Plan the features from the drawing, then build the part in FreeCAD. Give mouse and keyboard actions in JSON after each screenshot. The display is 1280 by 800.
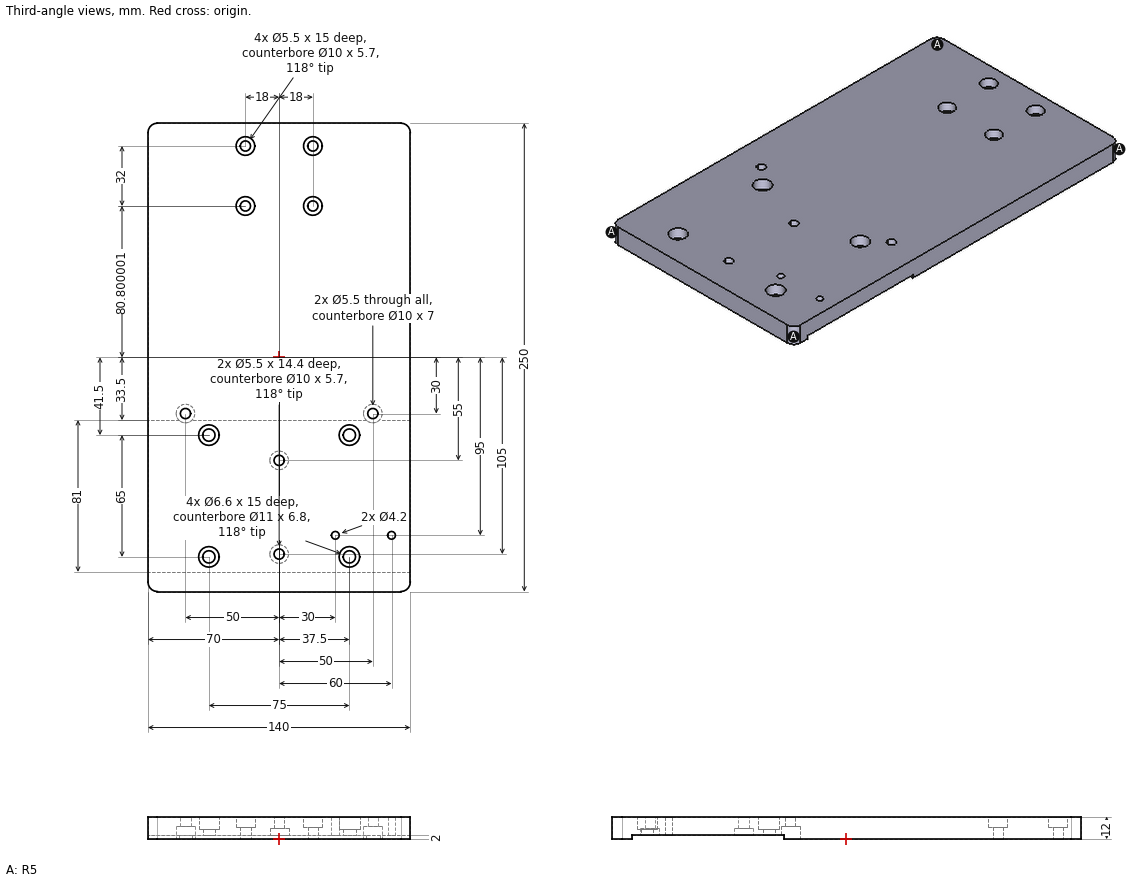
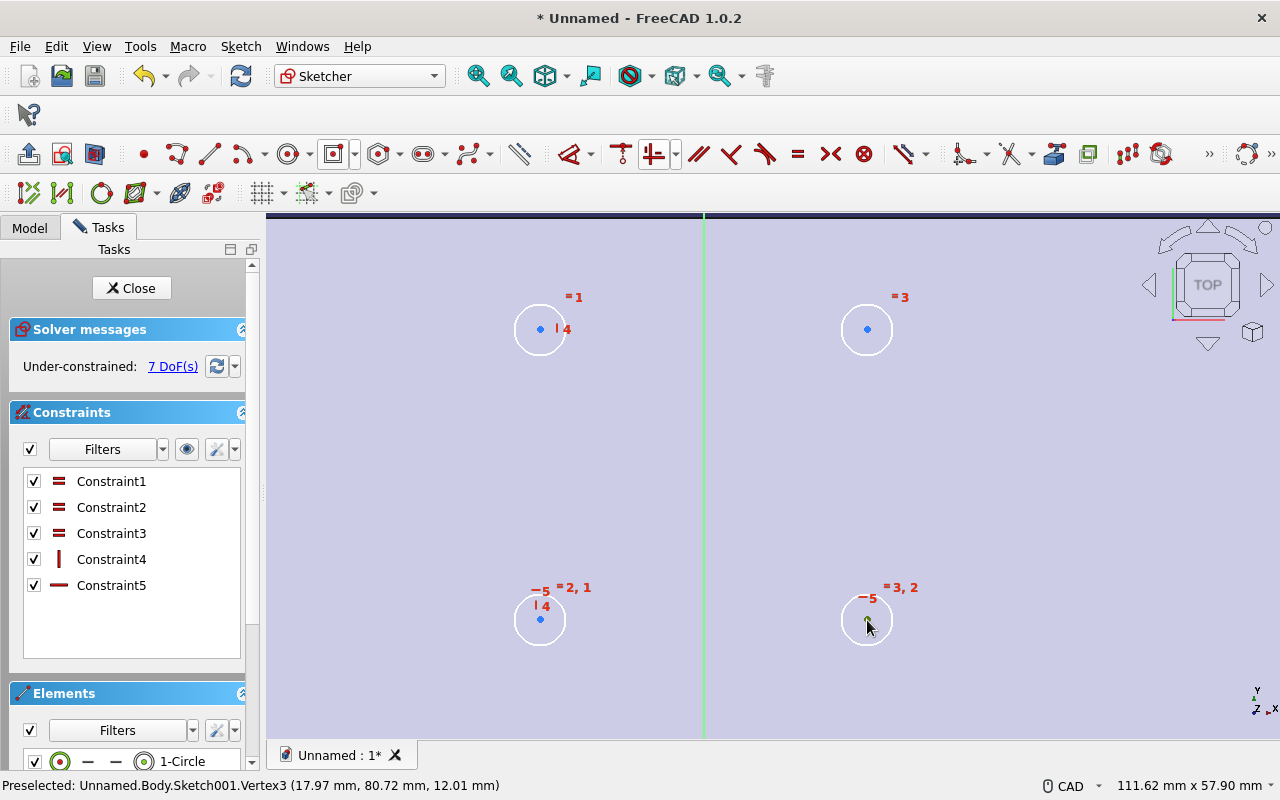
{"action": "left_click", "coordinate": [867, 330]}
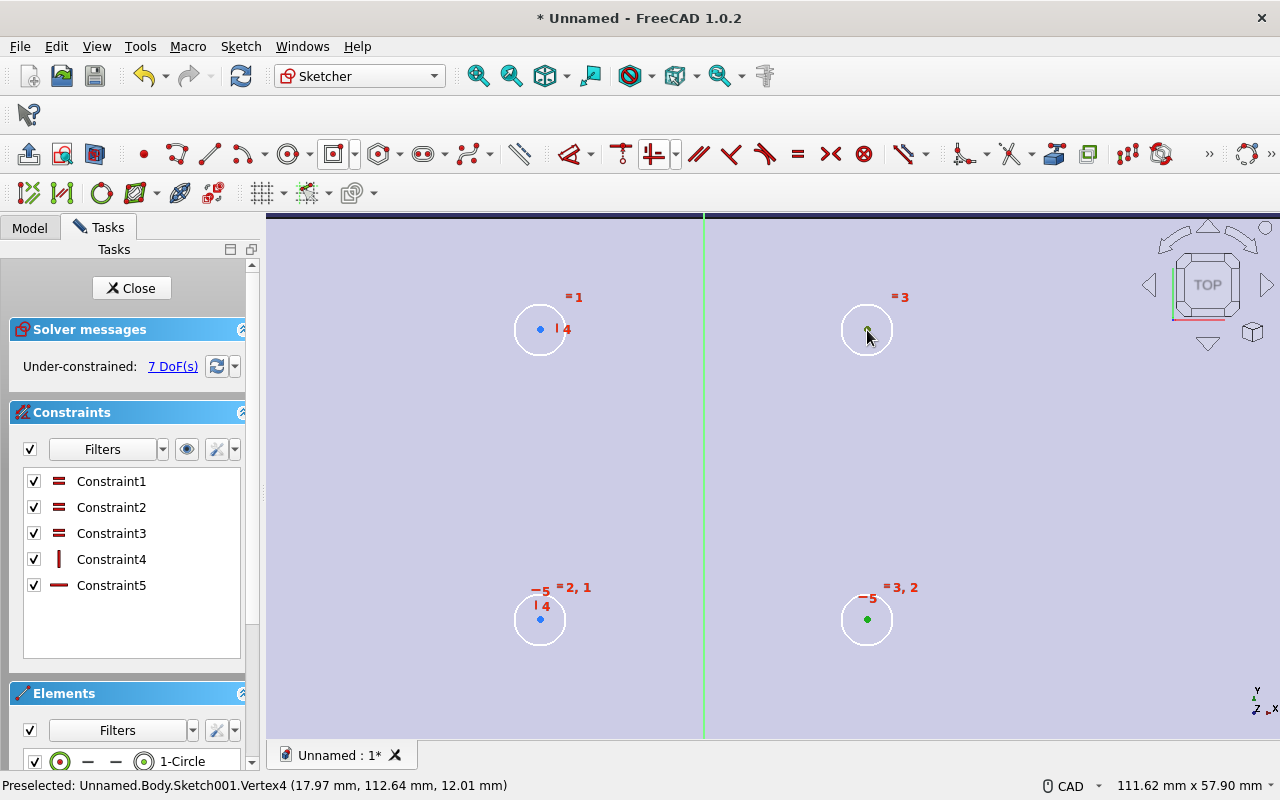
{"action": "left_click", "coordinate": [676, 154]}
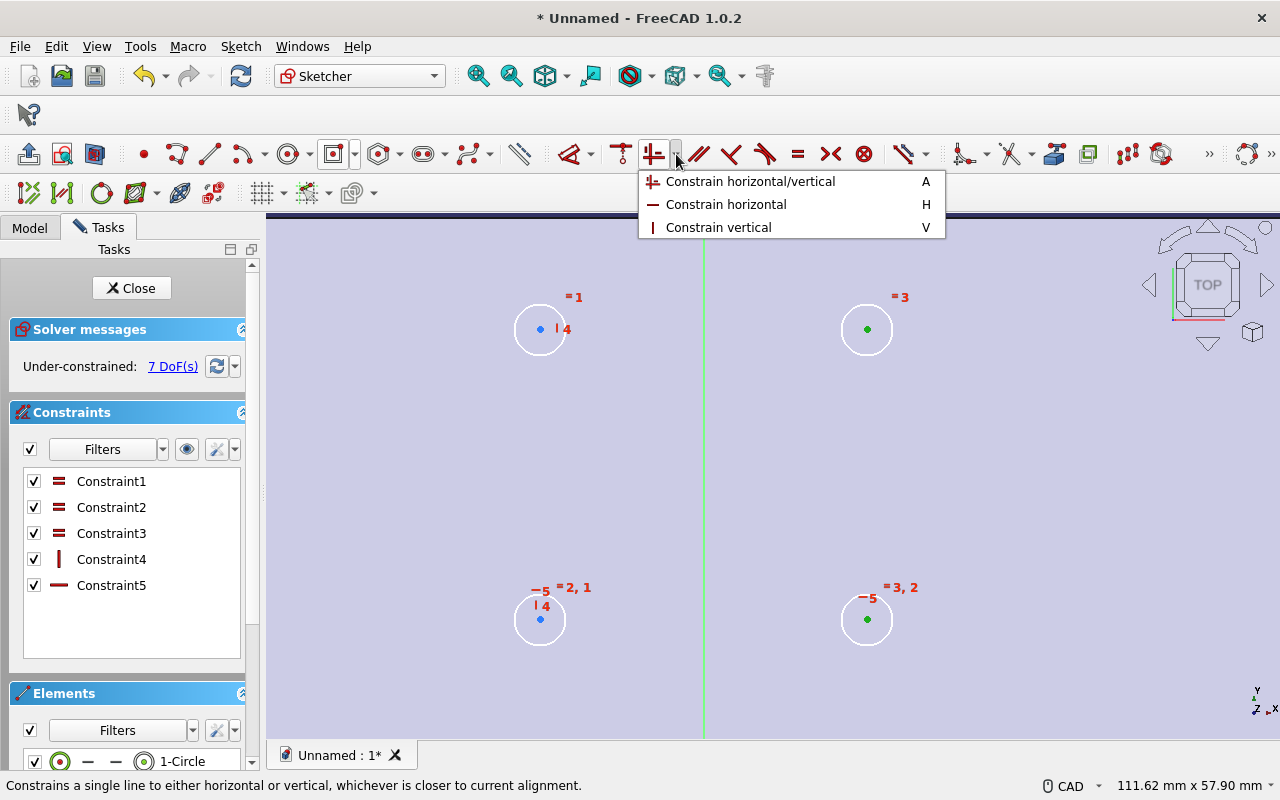
{"action": "left_click", "coordinate": [792, 228]}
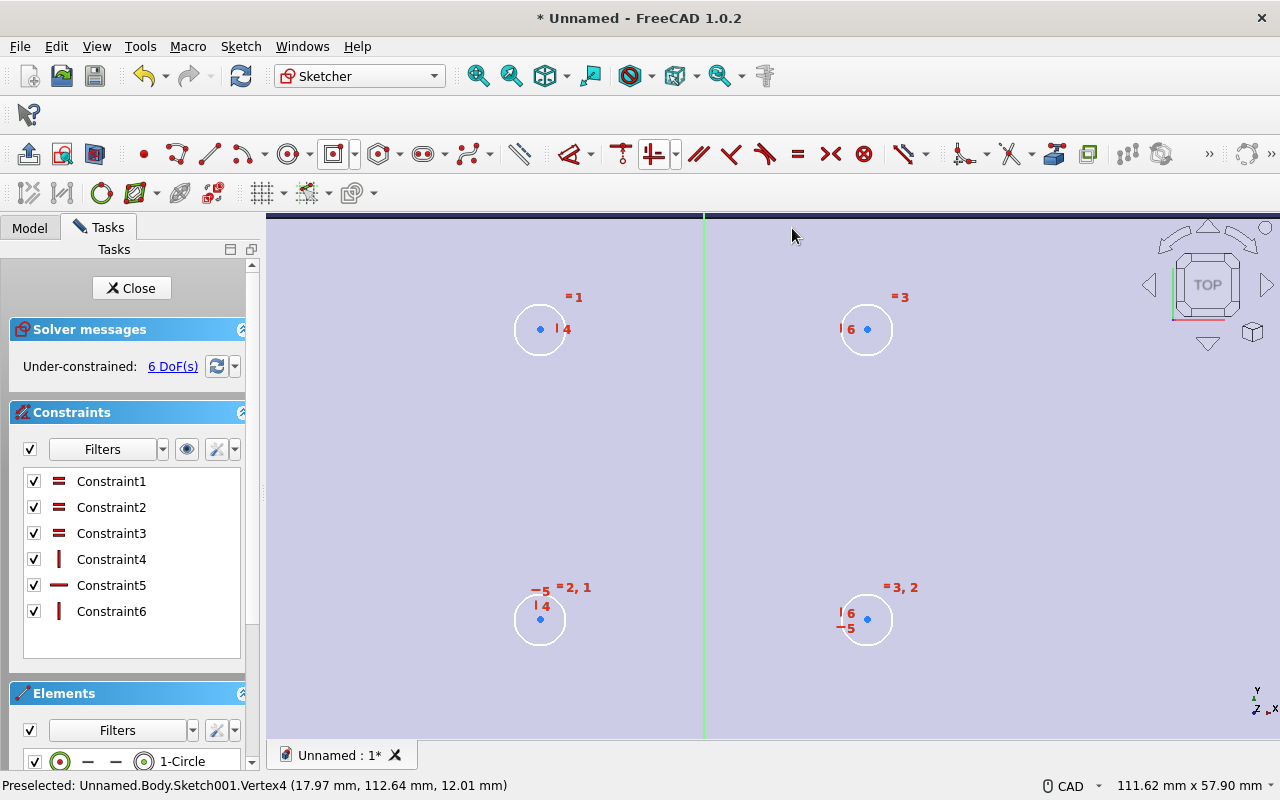
{"action": "left_click", "coordinate": [540, 330]}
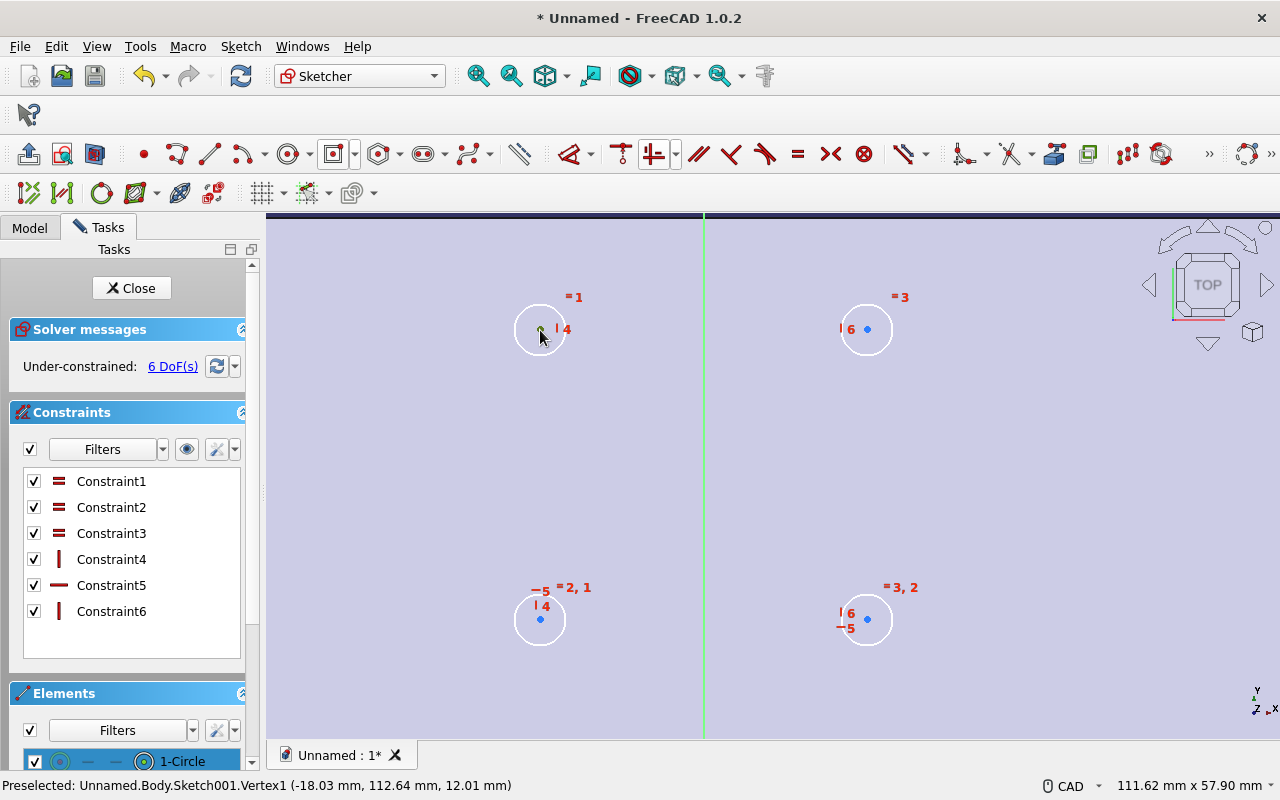
{"action": "left_click", "coordinate": [867, 330]}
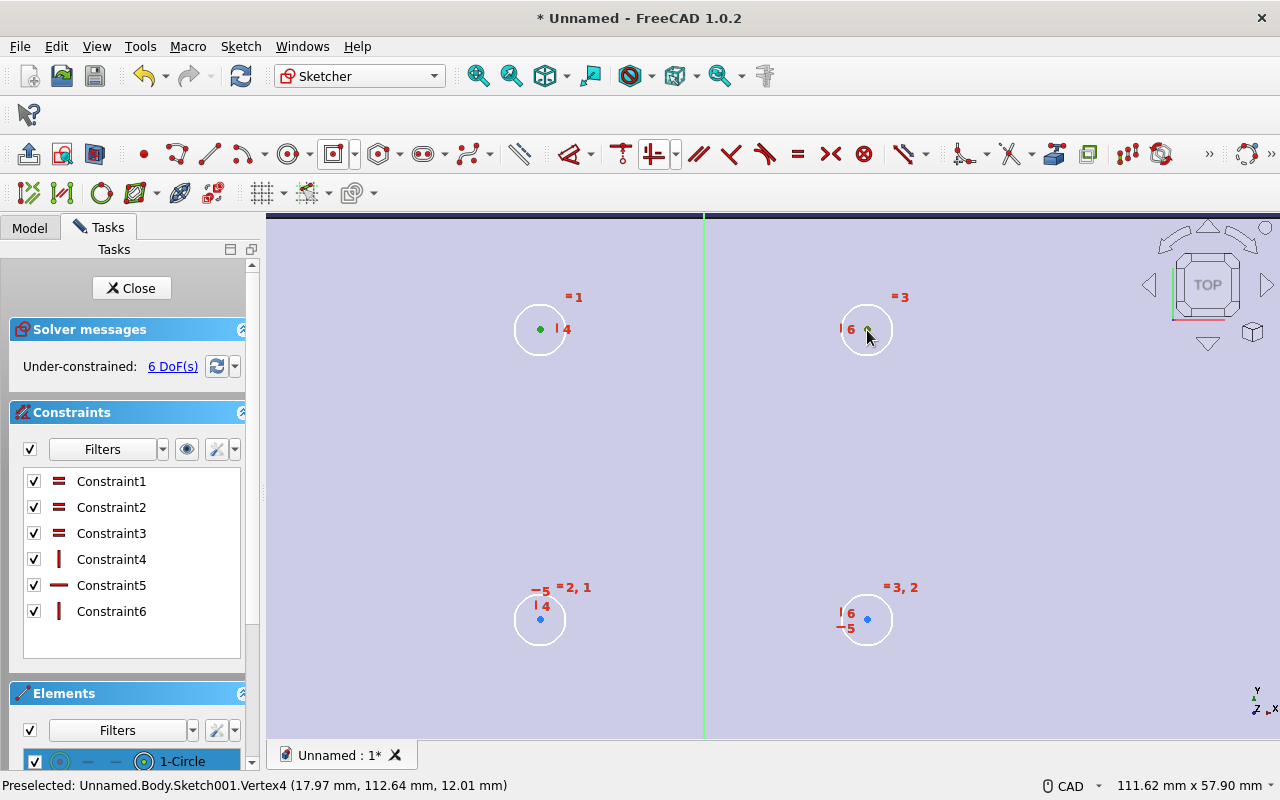
{"action": "key", "text": "h"}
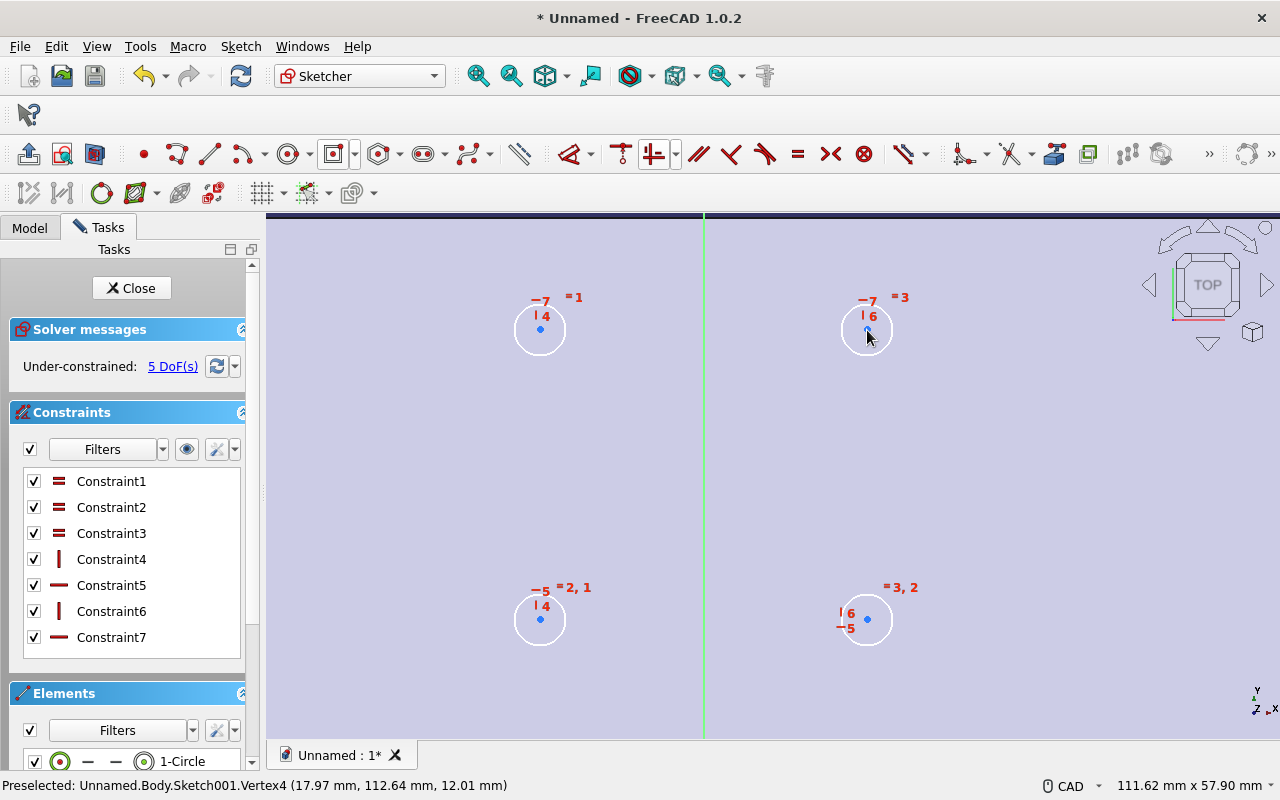
{"action": "left_click", "coordinate": [558, 312]}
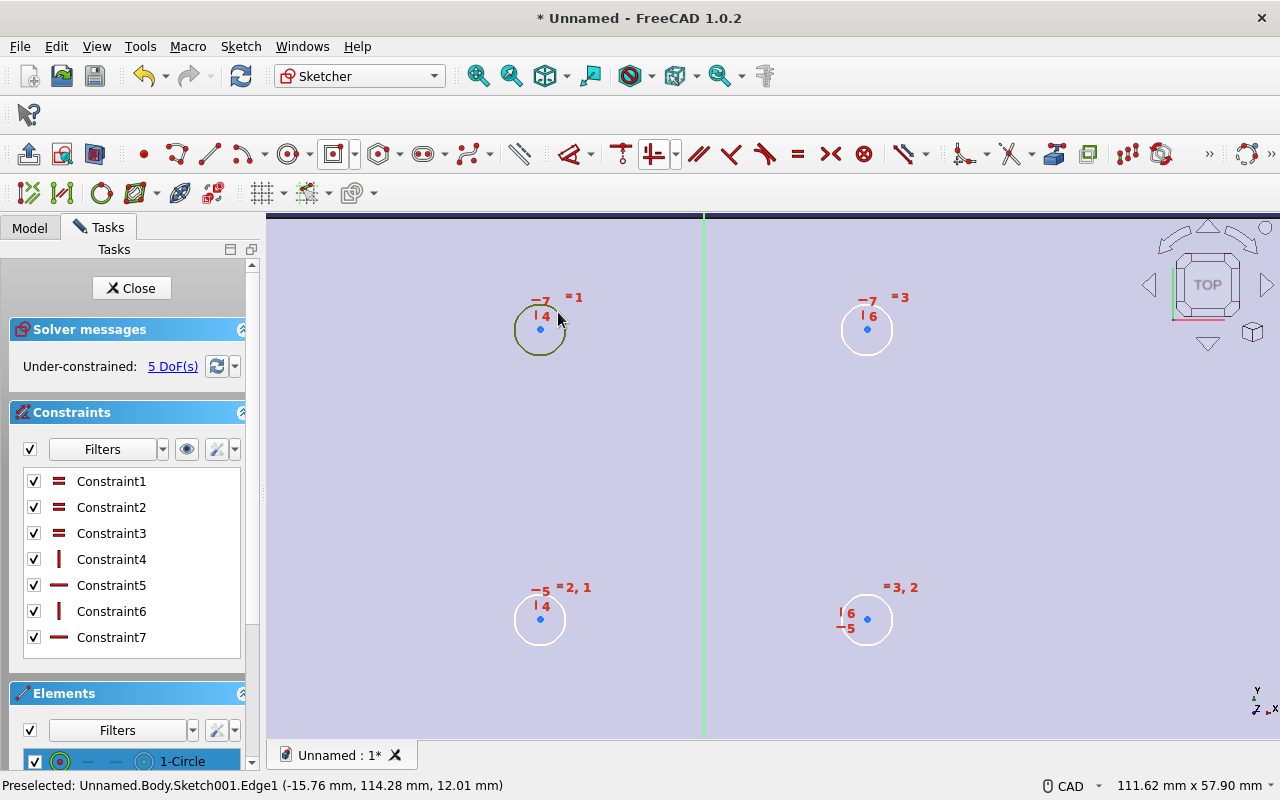
{"action": "key", "text": "k o"}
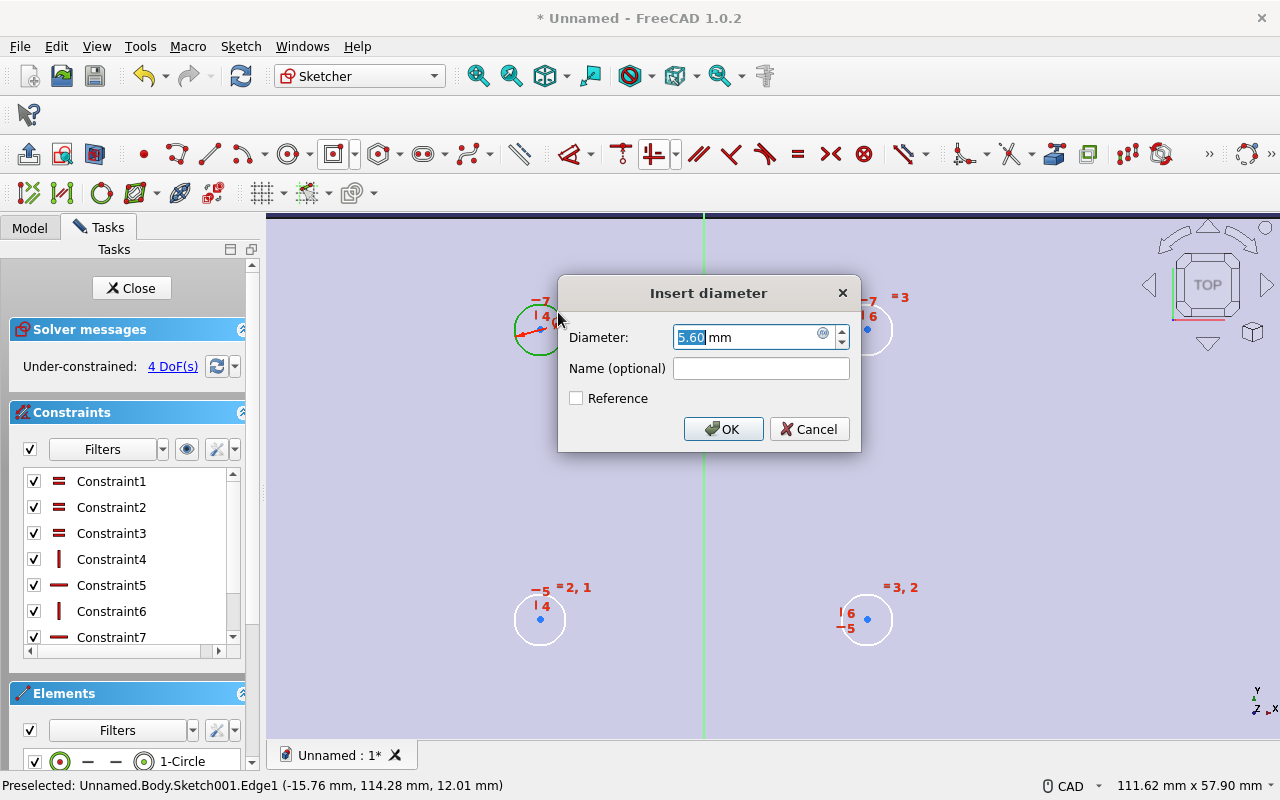
{"action": "type", "text": "5.5"}
{"action": "key", "text": "Return"}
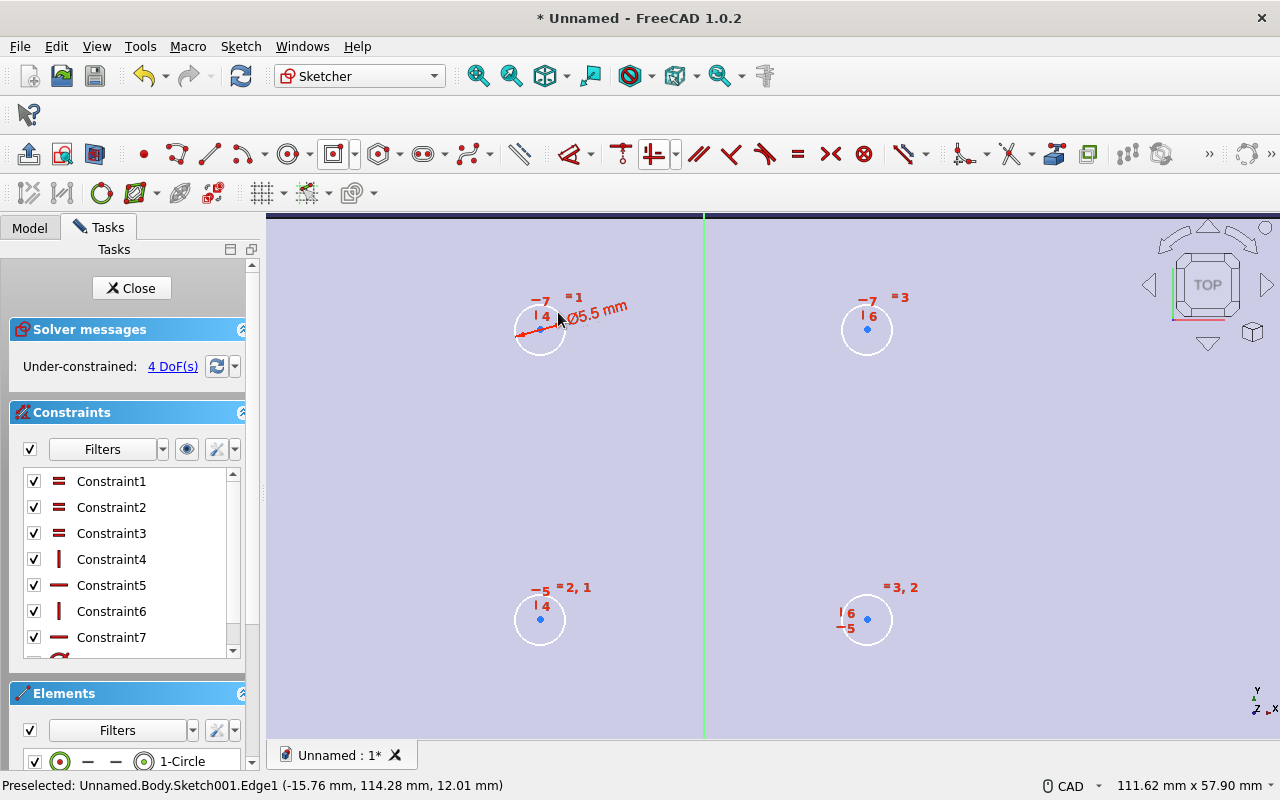
{"action": "left_click", "coordinate": [540, 330]}